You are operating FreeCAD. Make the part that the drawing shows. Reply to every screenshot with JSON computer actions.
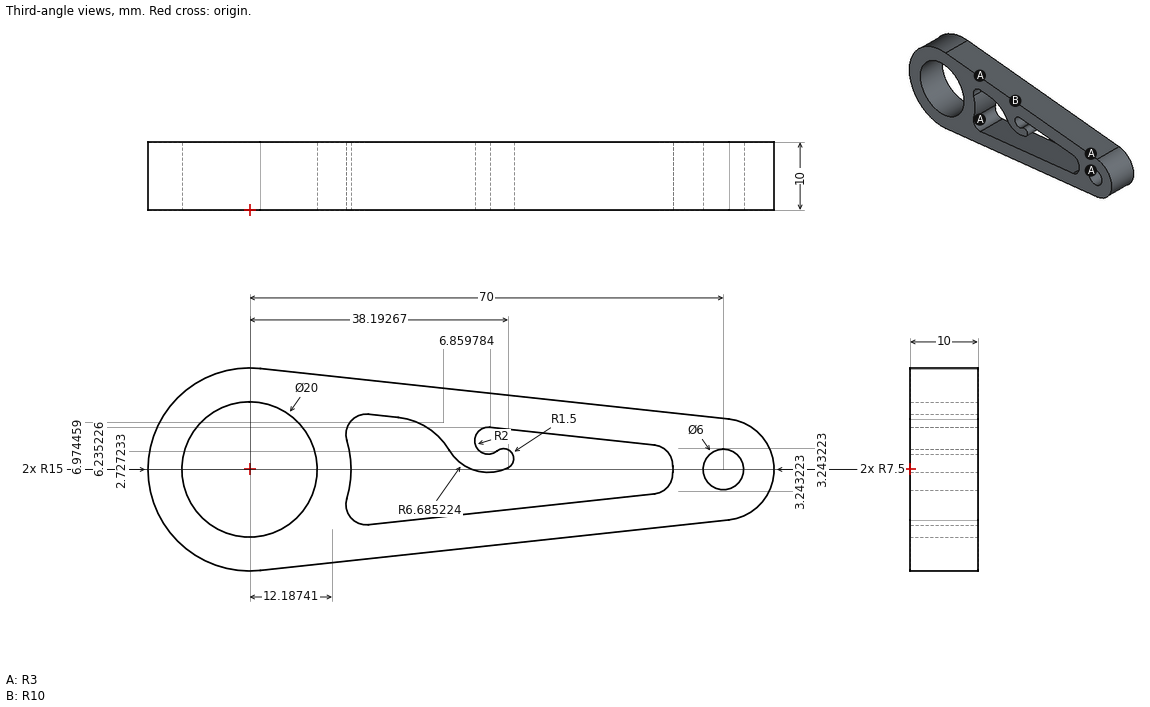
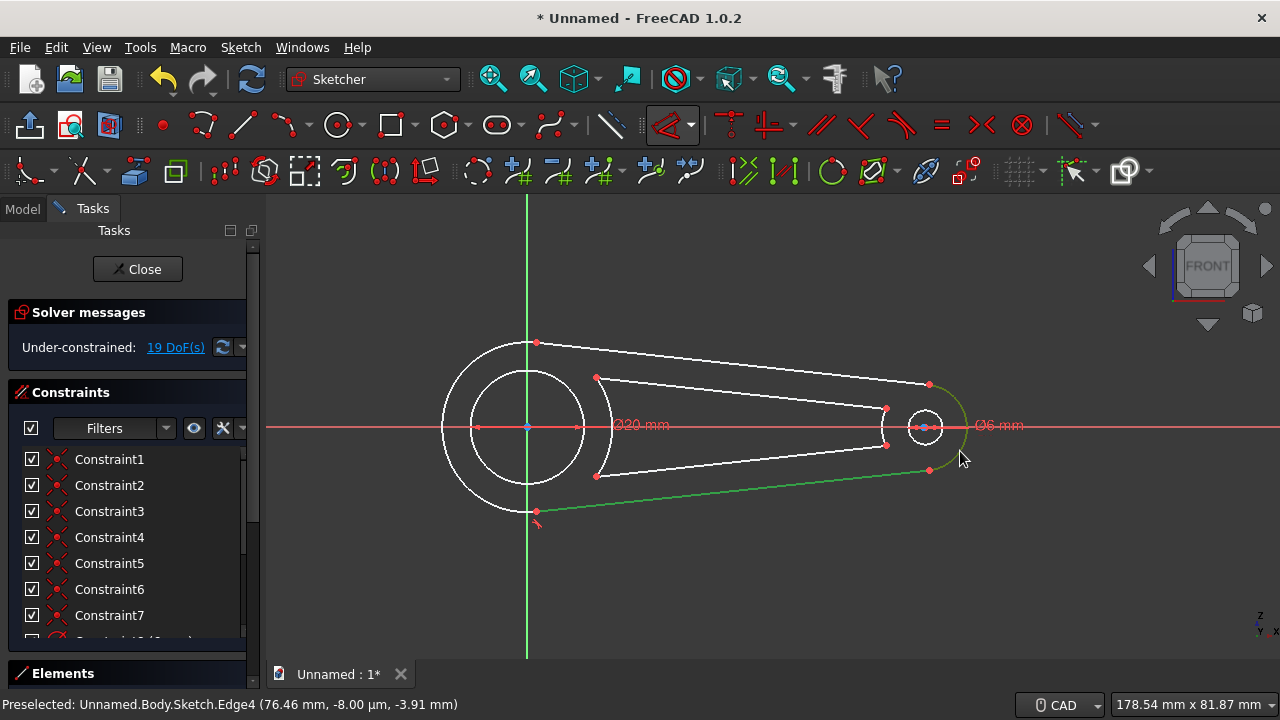
{"action": "key", "text": "t"}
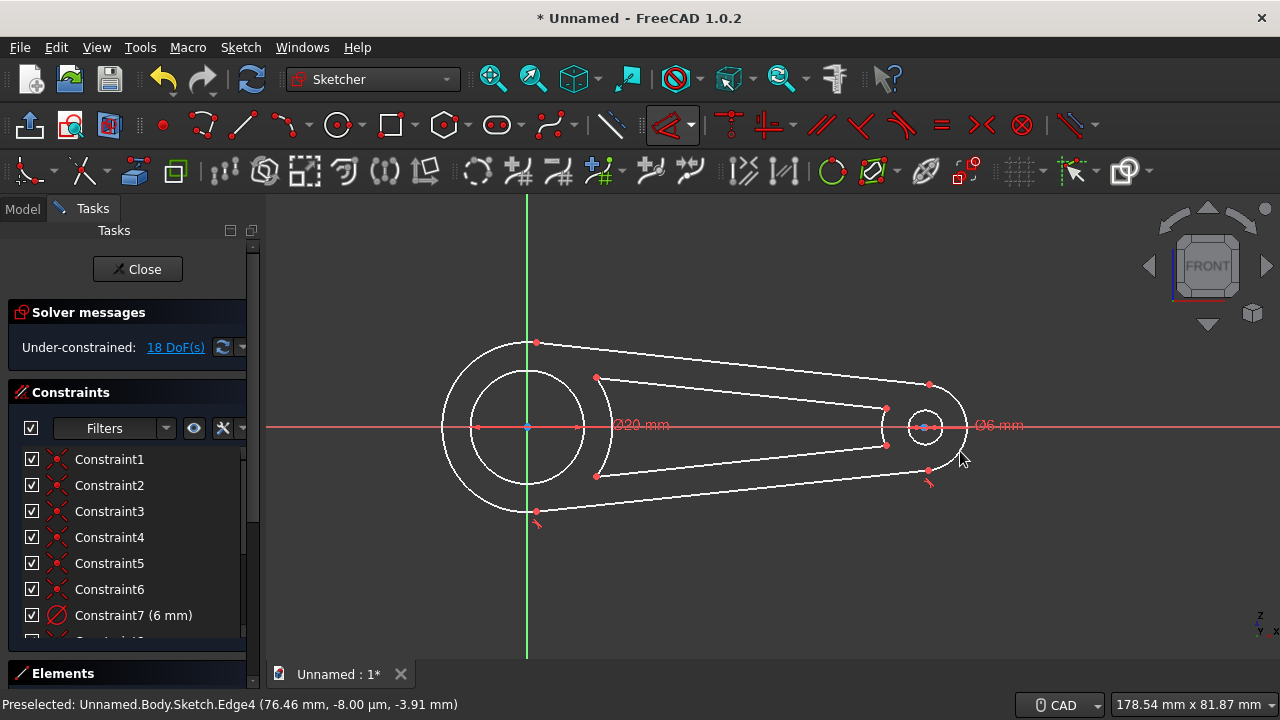
{"action": "left_click", "coordinate": [654, 355]}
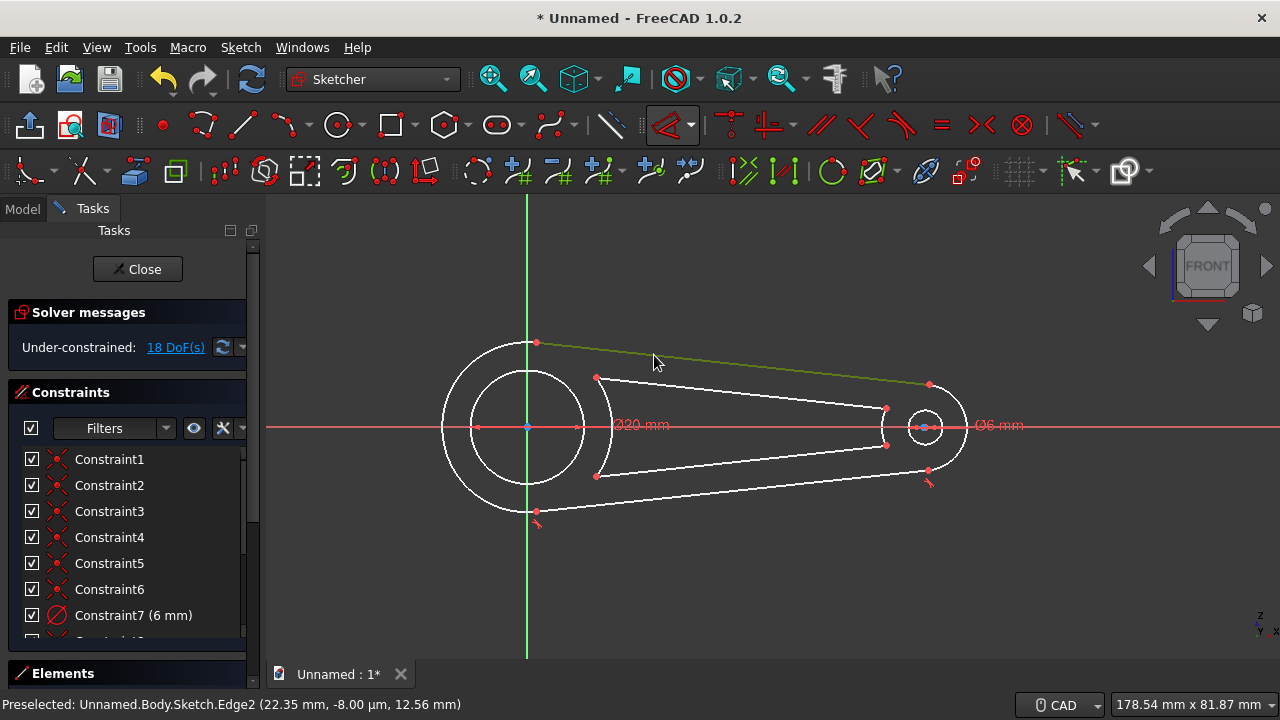
{"action": "left_click", "coordinate": [461, 374]}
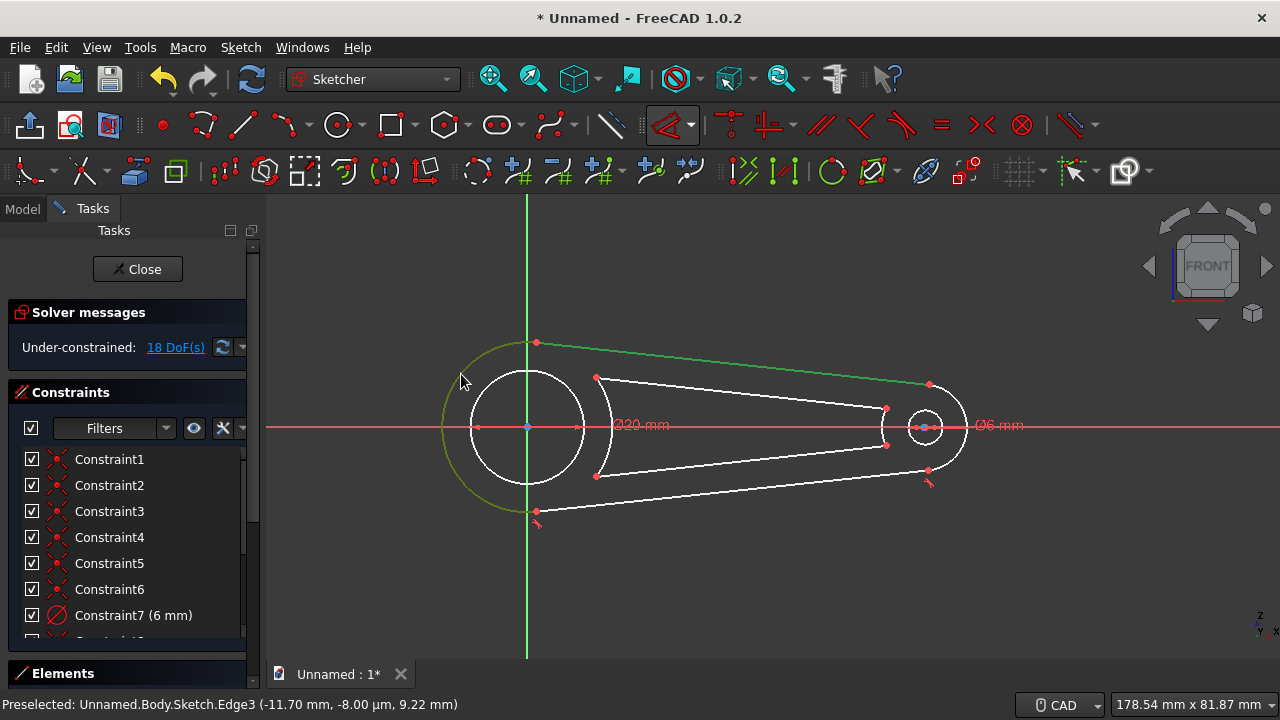
{"action": "left_click", "coordinate": [902, 126]}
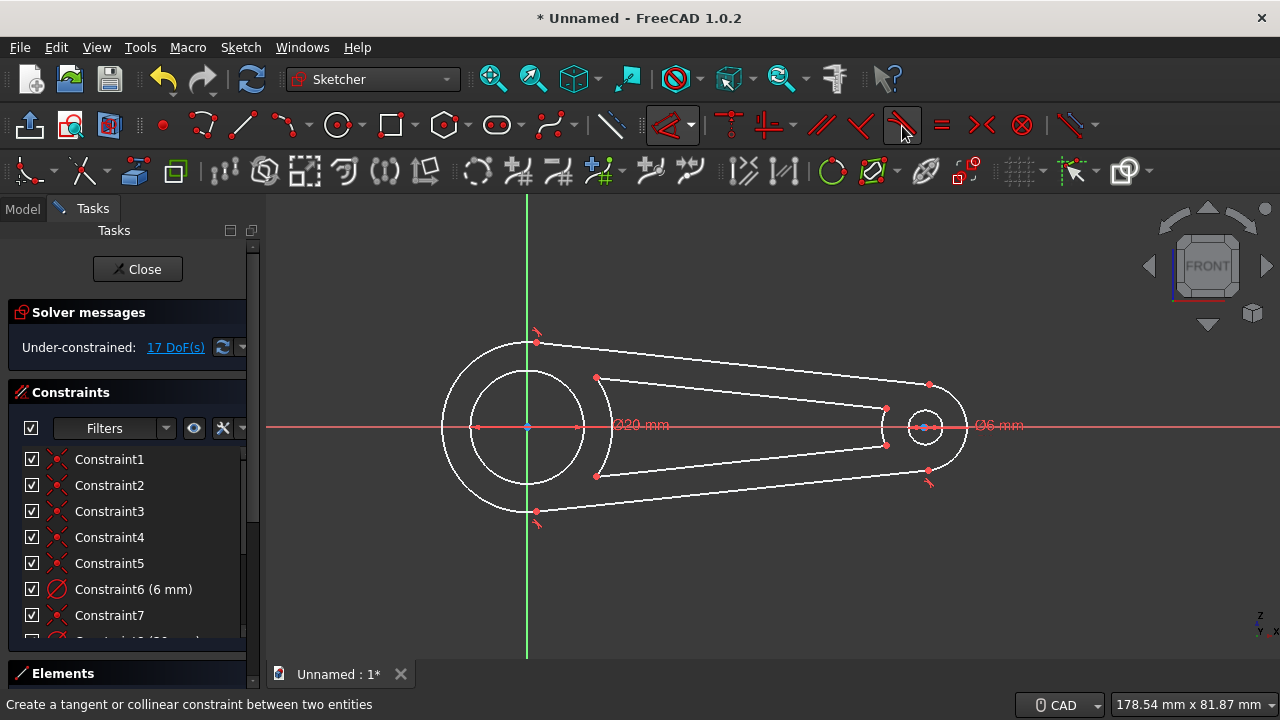
{"action": "left_click", "coordinate": [654, 355]}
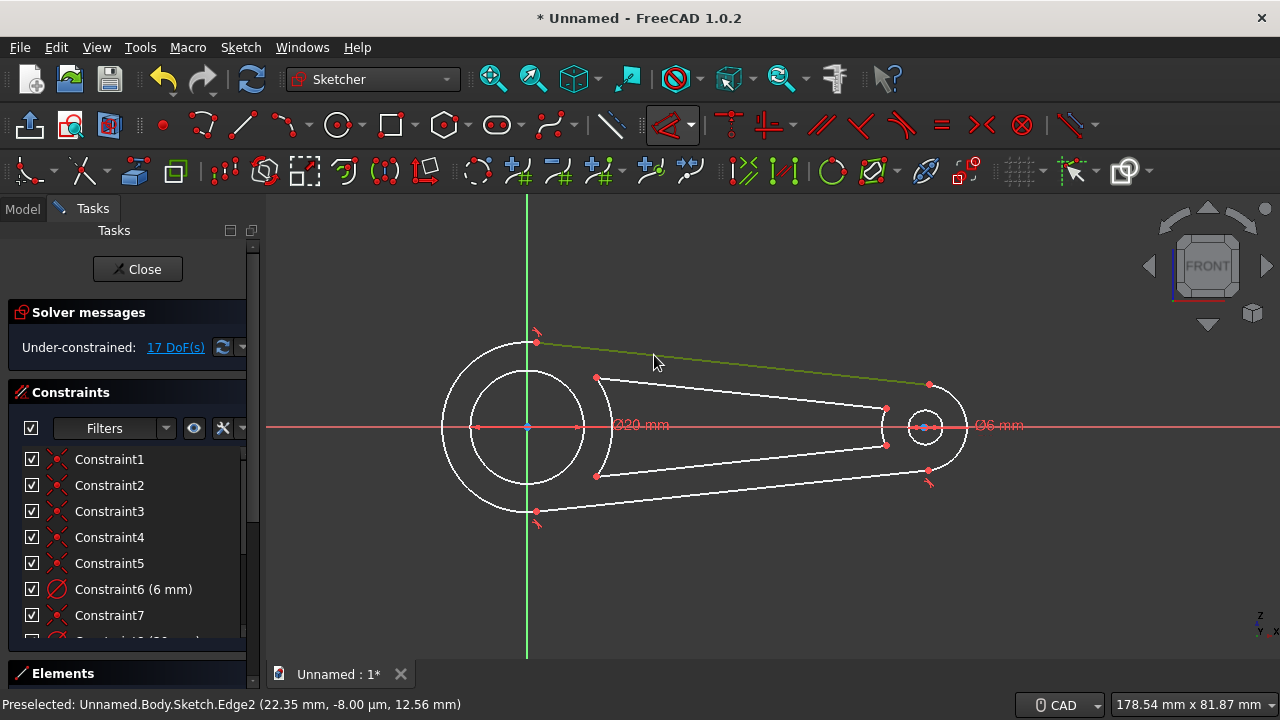
{"action": "left_click", "coordinate": [960, 452]}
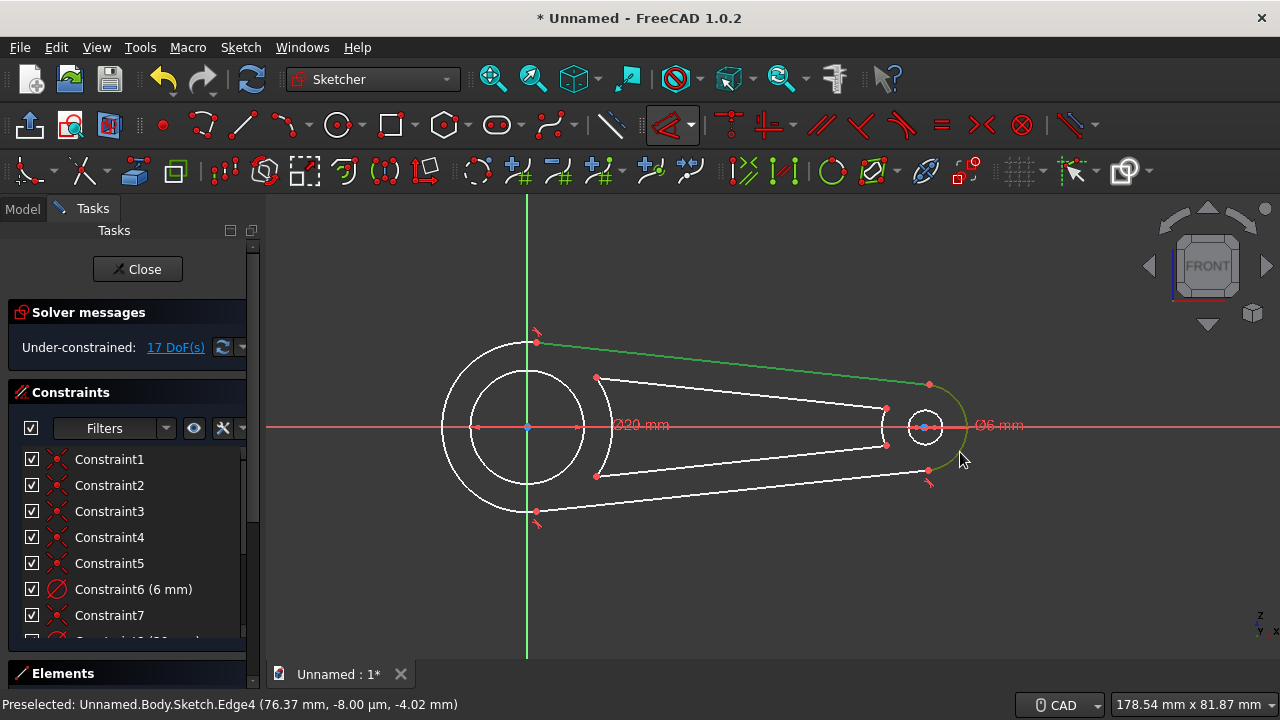
{"action": "key", "text": "t"}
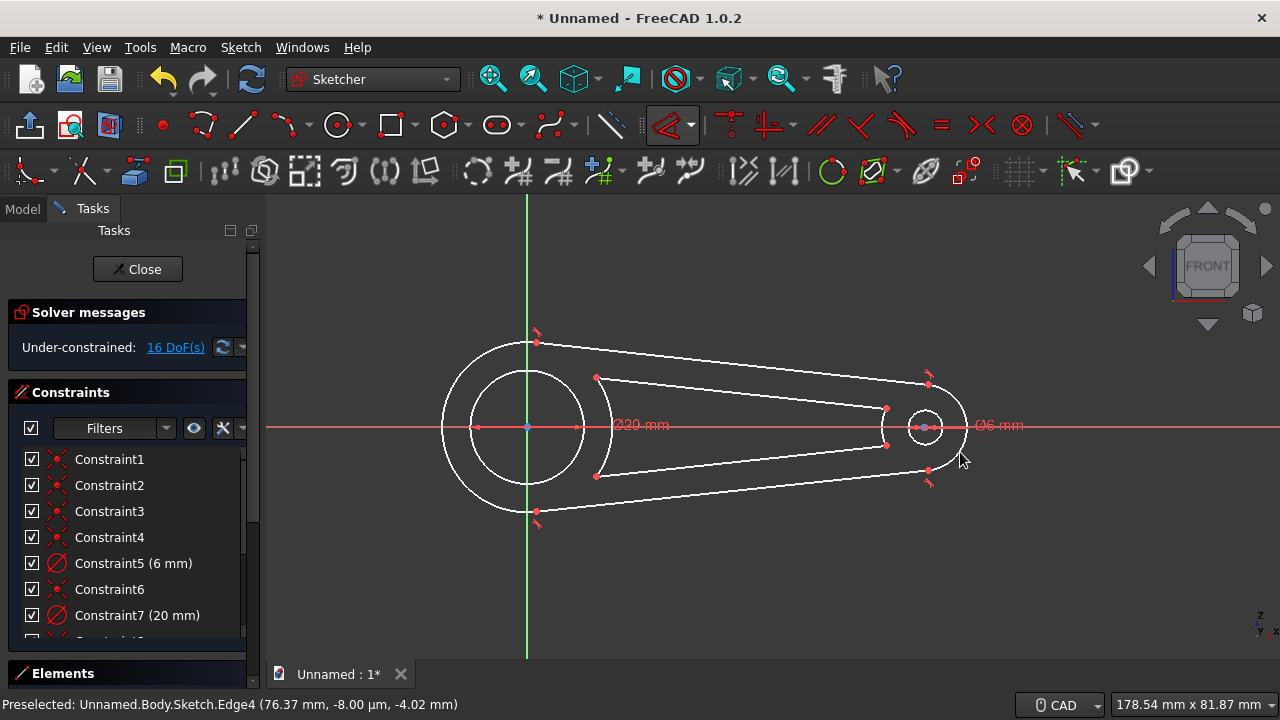
{"action": "left_click", "coordinate": [937, 415]}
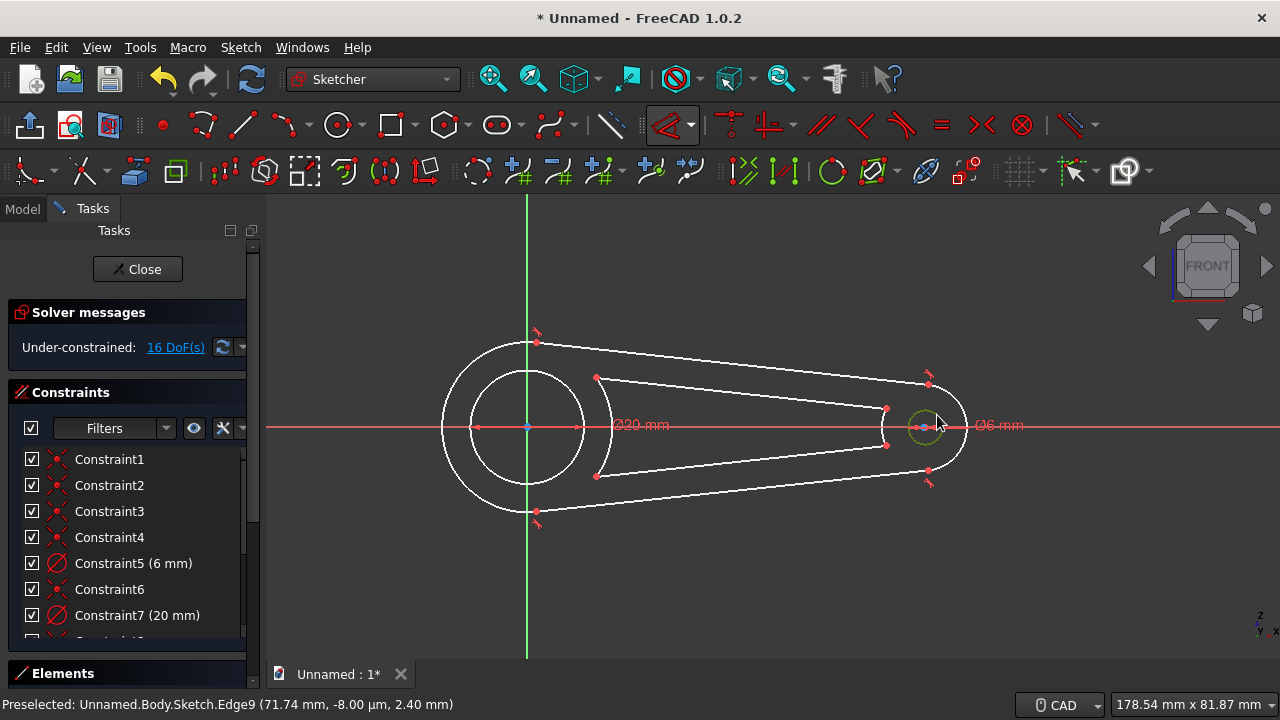
{"action": "left_click", "coordinate": [960, 452]}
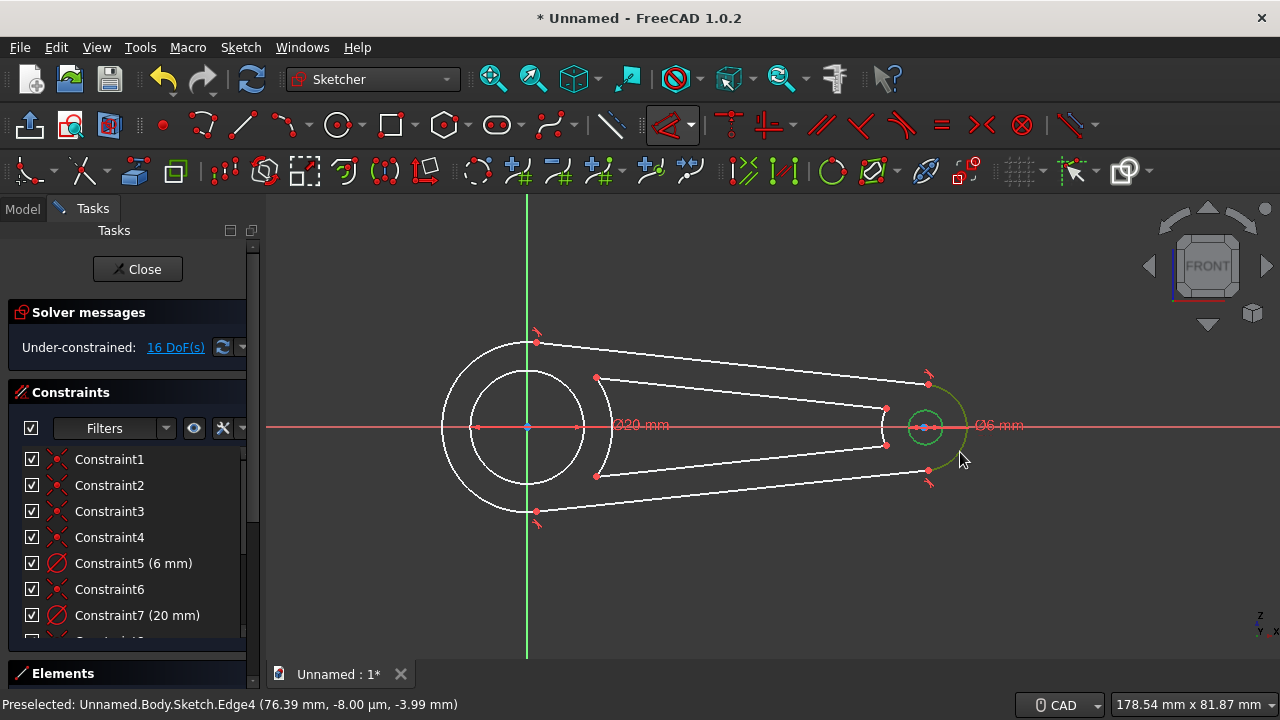
{"action": "left_click", "coordinate": [730, 126]}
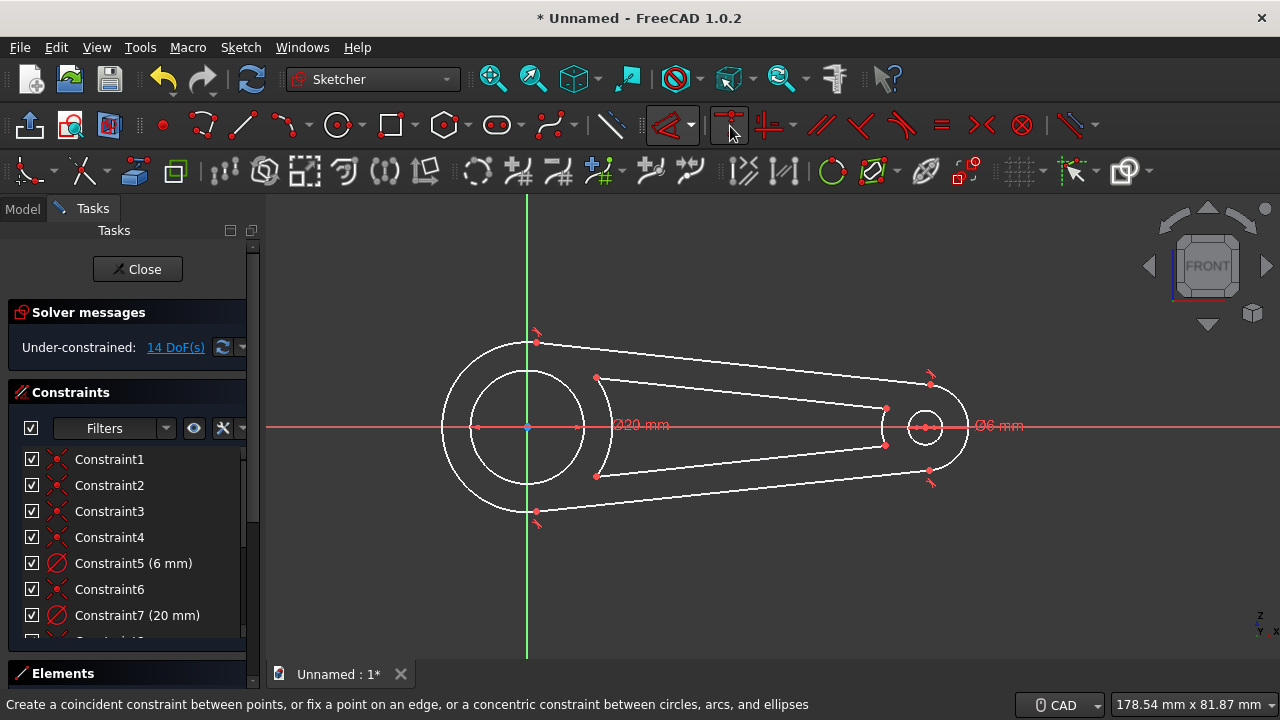
{"action": "left_click", "coordinate": [567, 387]}